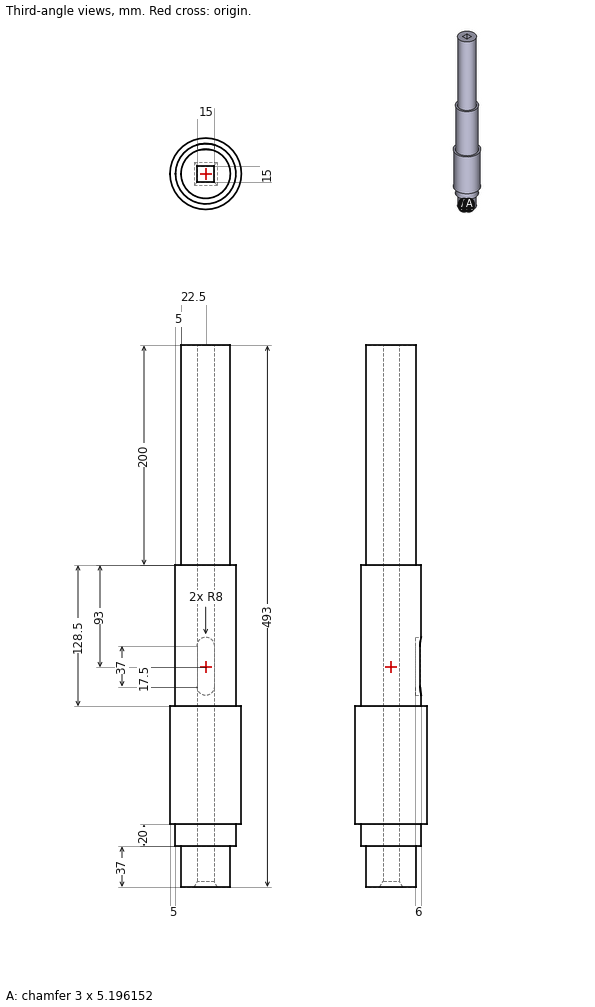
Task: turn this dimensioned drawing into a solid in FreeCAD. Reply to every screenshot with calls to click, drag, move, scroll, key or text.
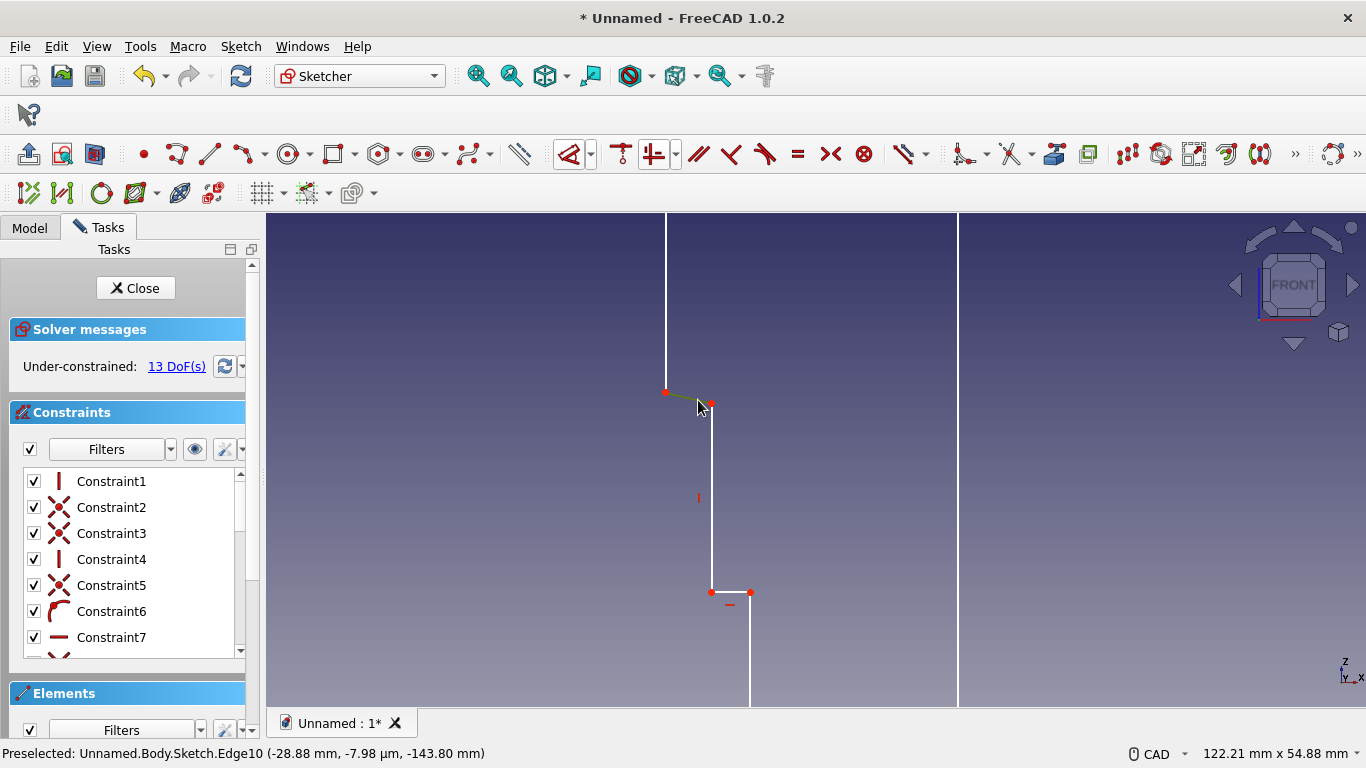
click(676, 154)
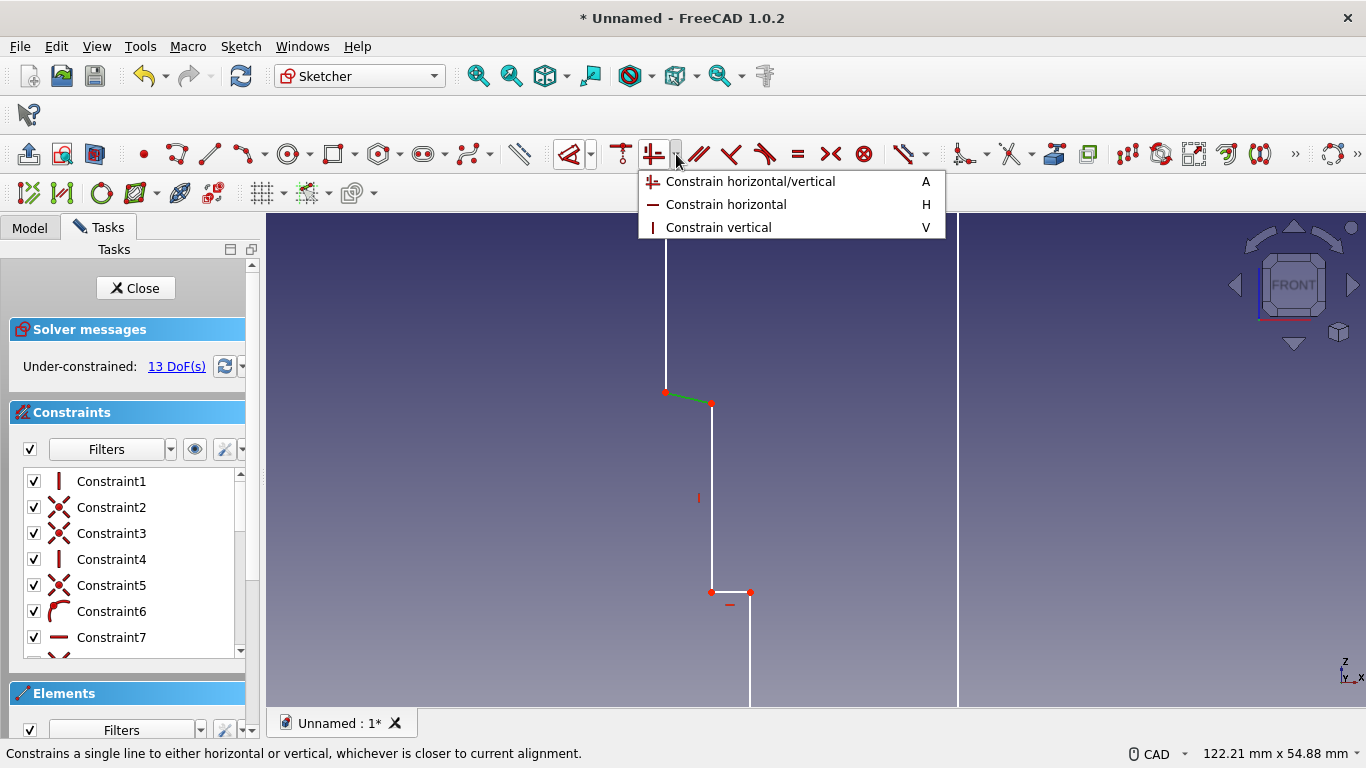
click(792, 204)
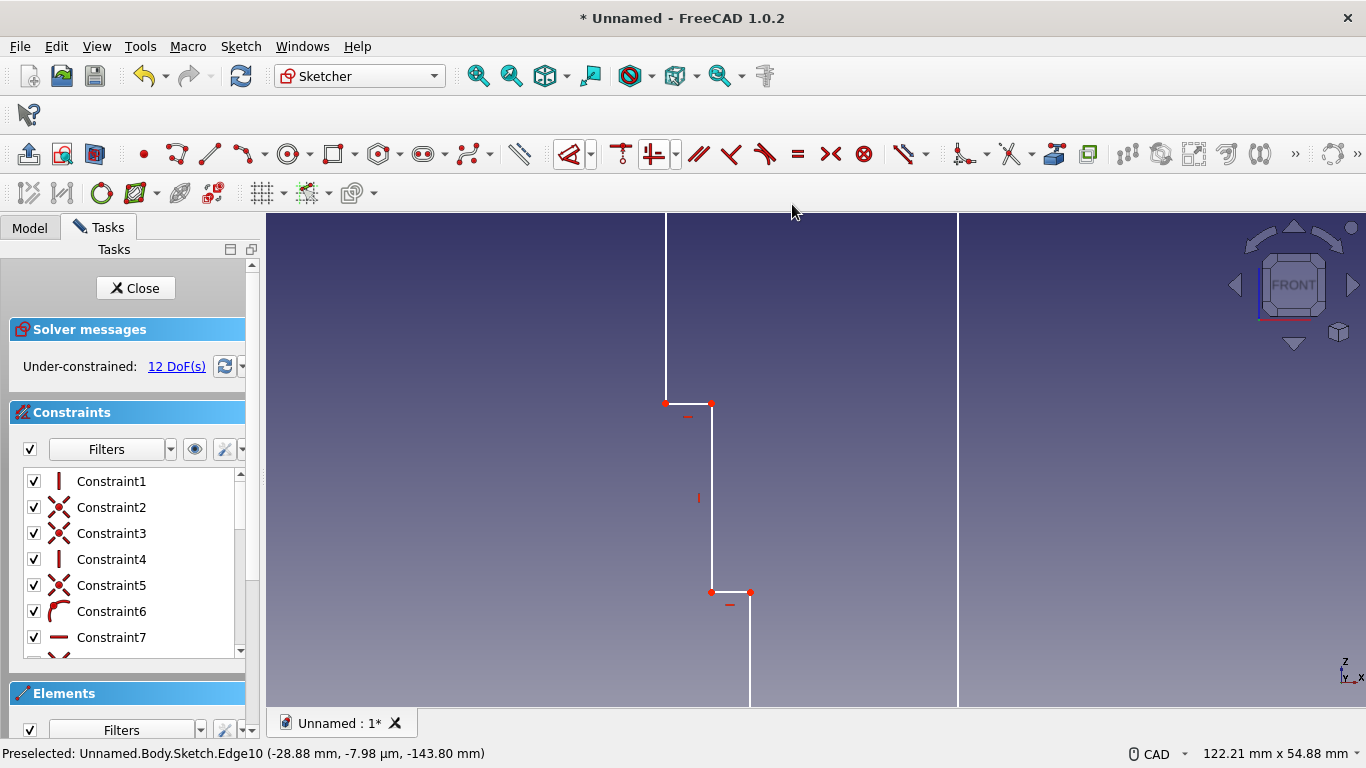
scroll(742, 602, down, 13)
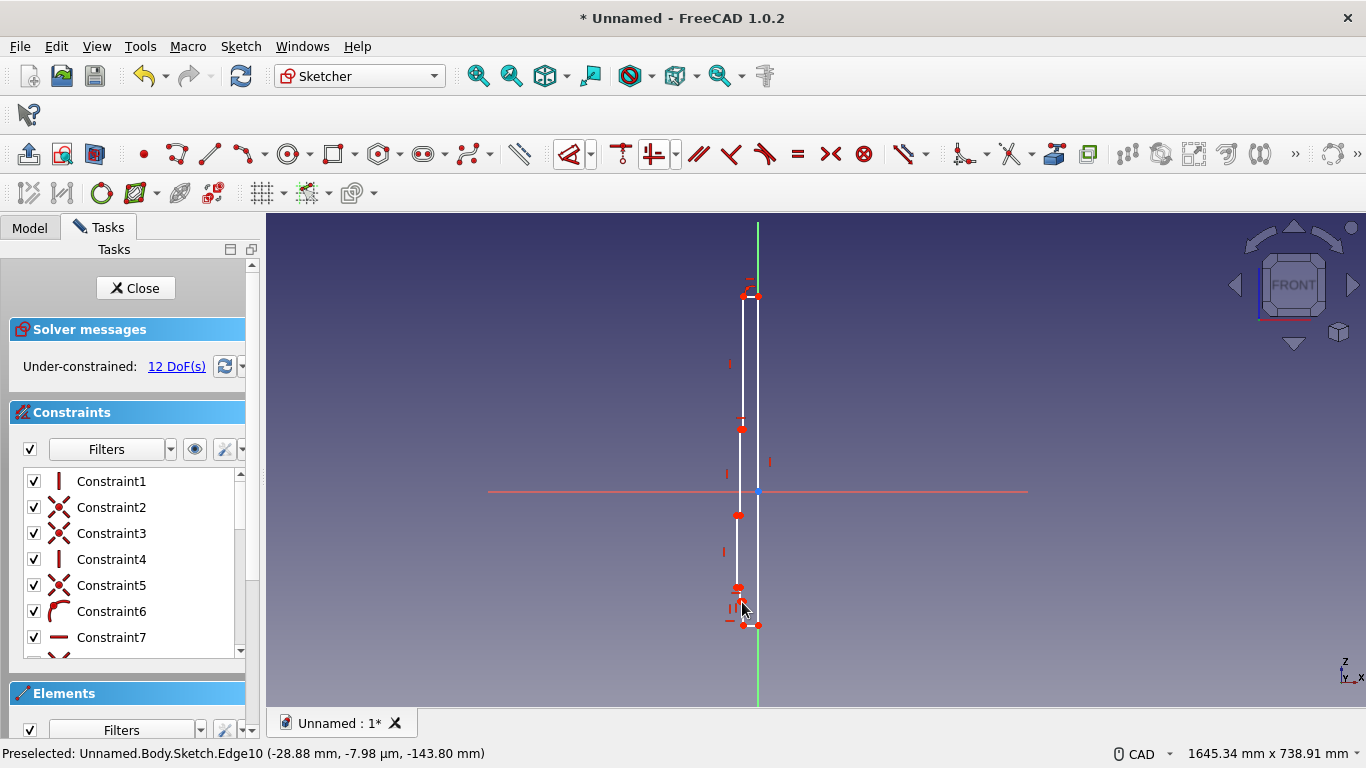
scroll(738, 516, up, 14)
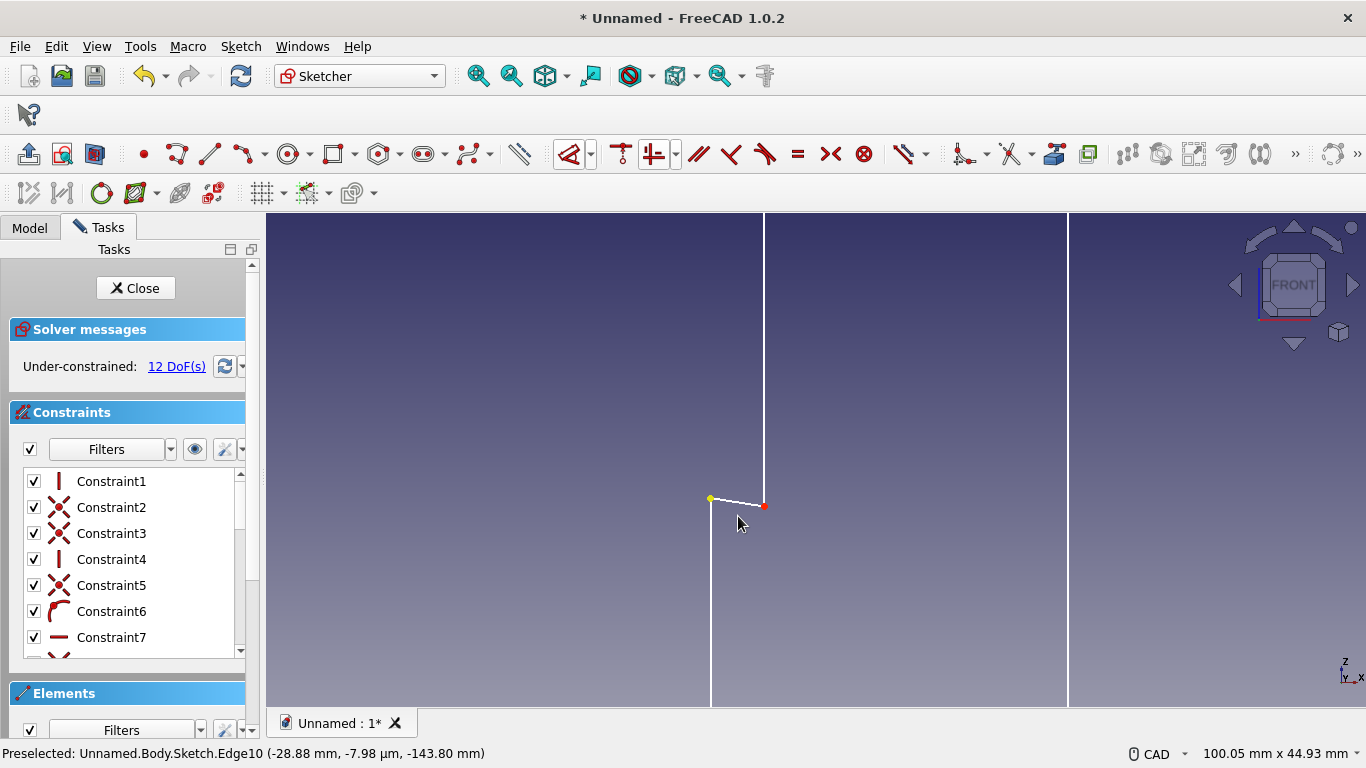
click(727, 501)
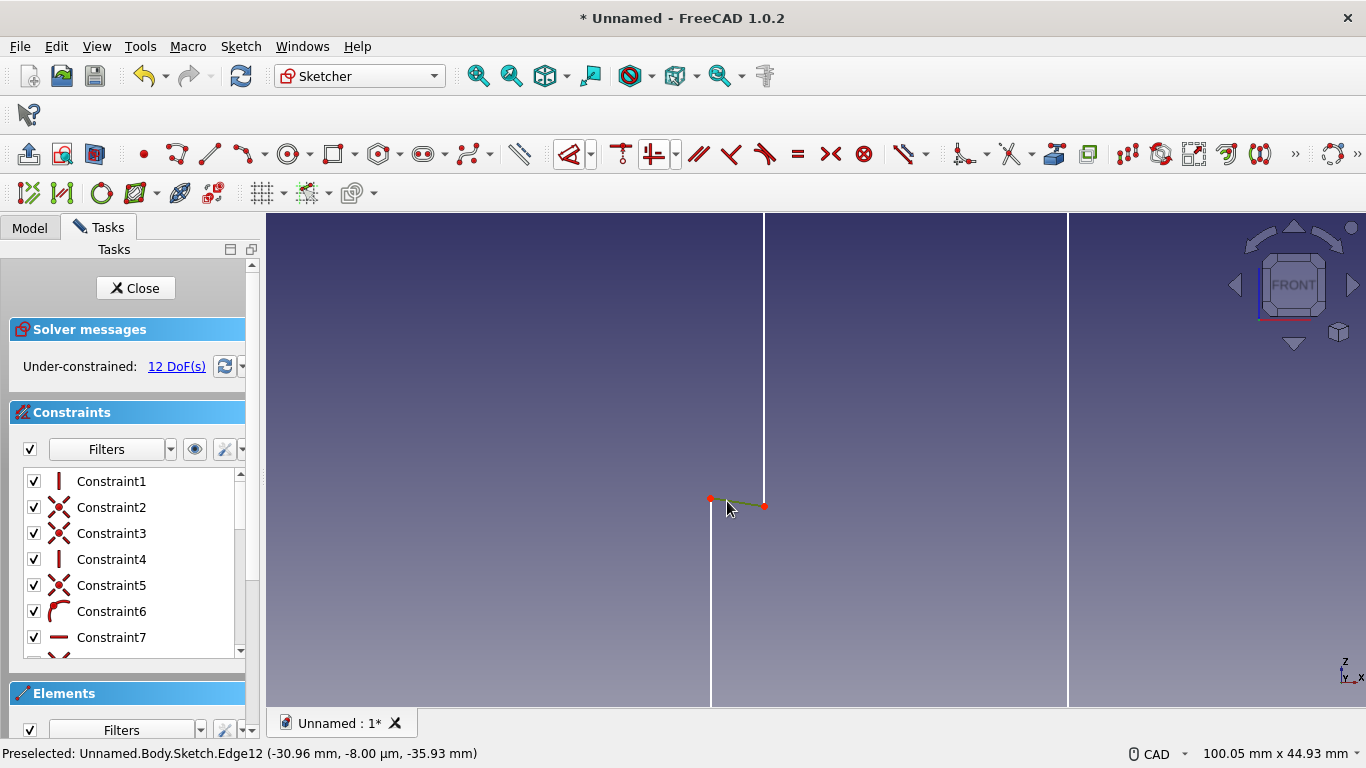
key(h)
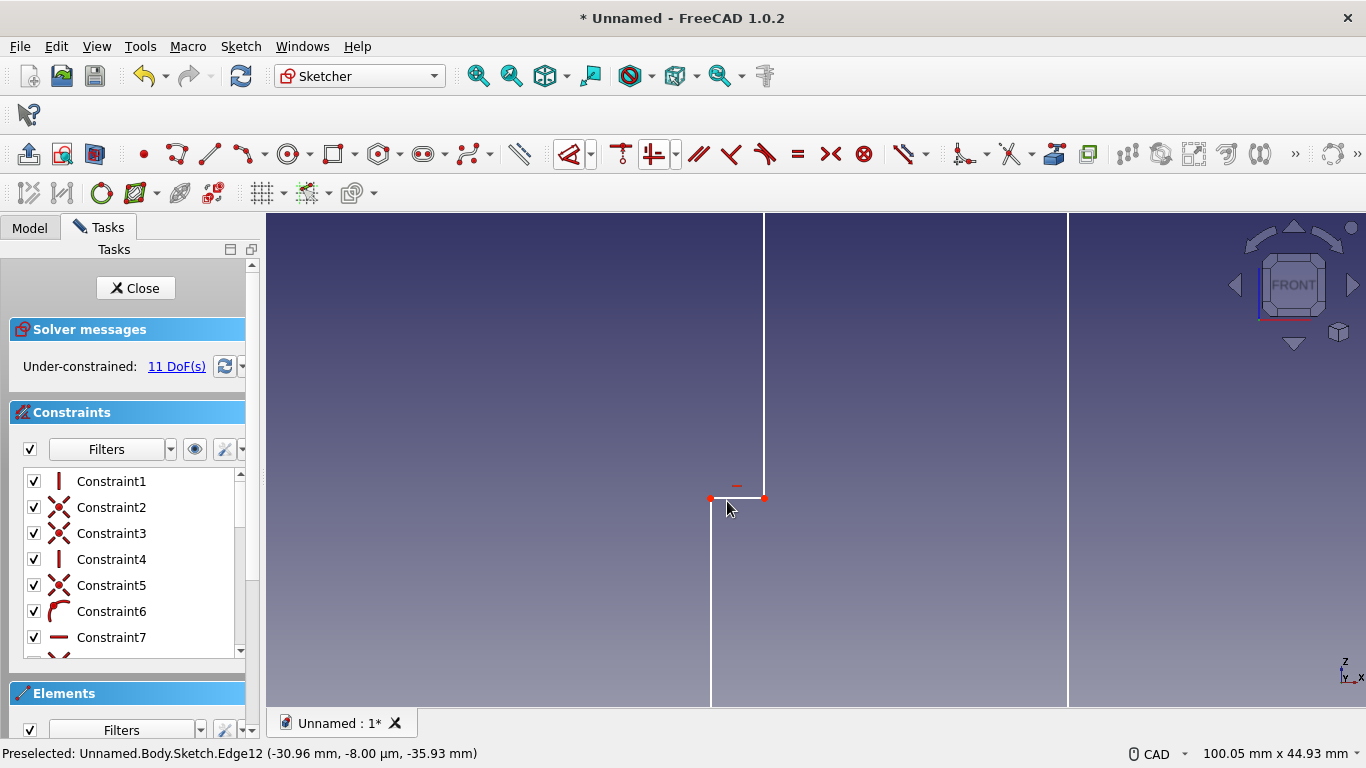
click(568, 154)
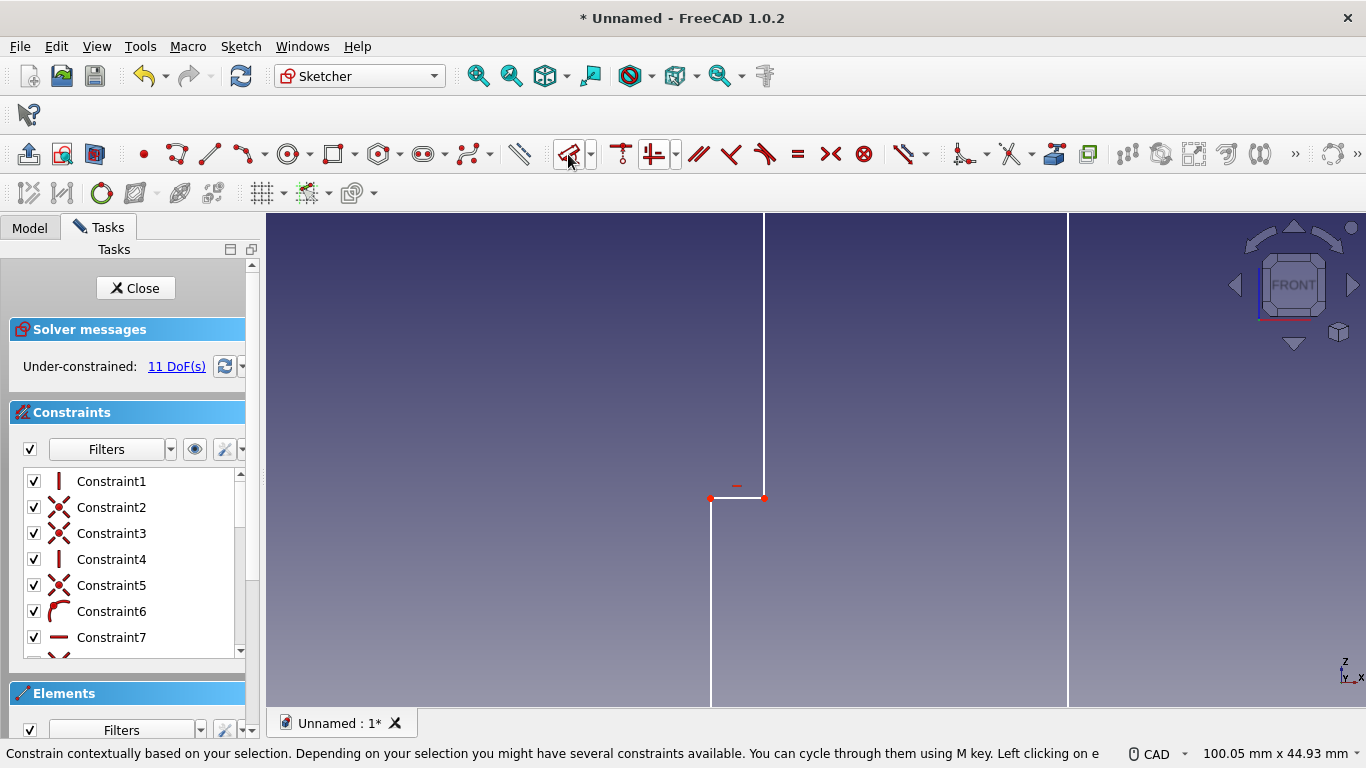
scroll(738, 516, down, 14)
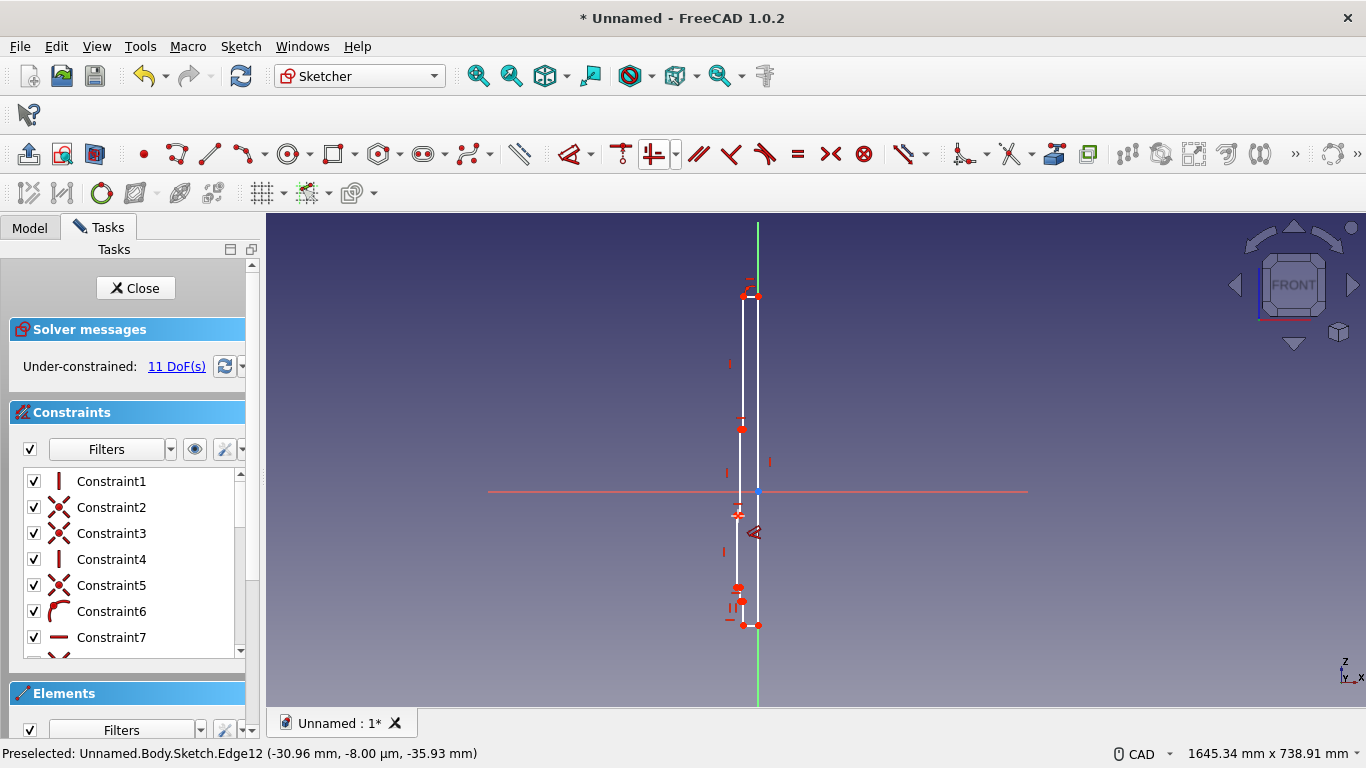
scroll(741, 430, up, 14)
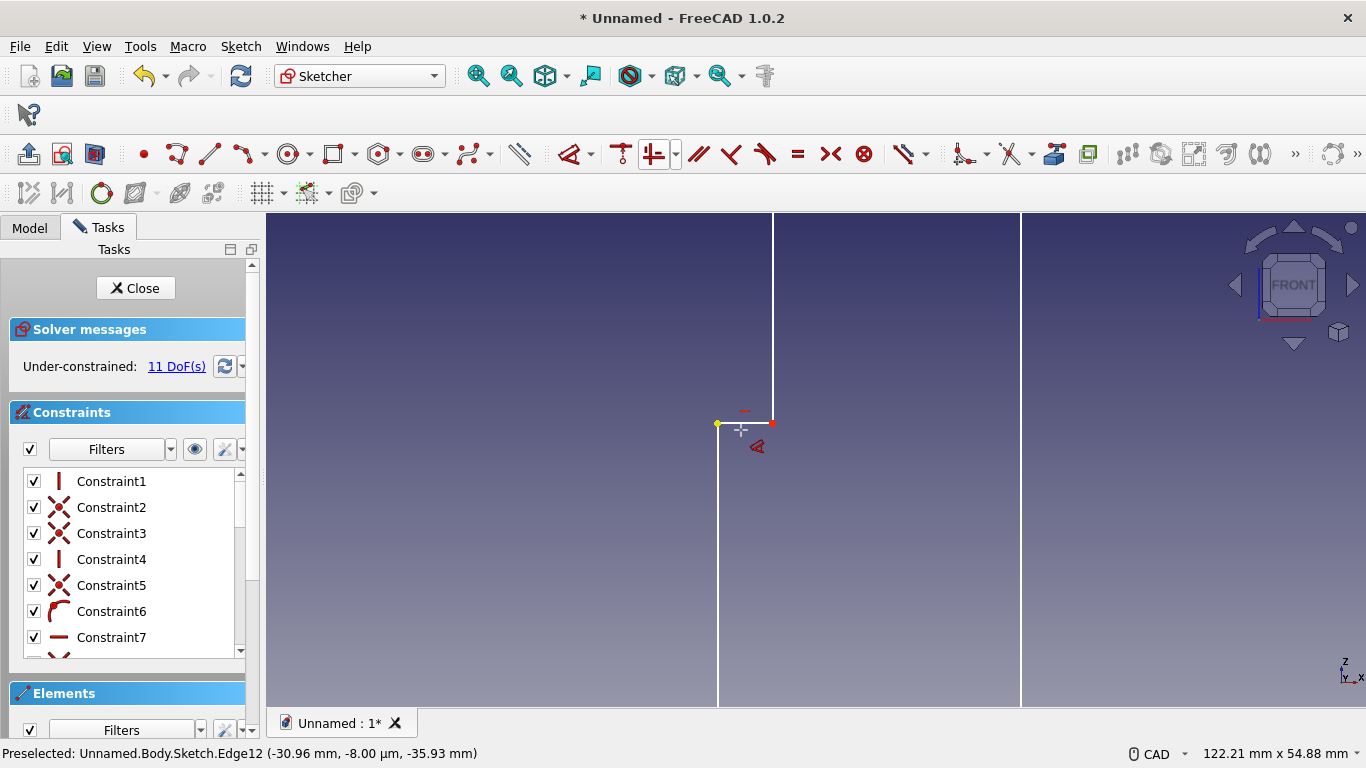
click(734, 423)
click(745, 389)